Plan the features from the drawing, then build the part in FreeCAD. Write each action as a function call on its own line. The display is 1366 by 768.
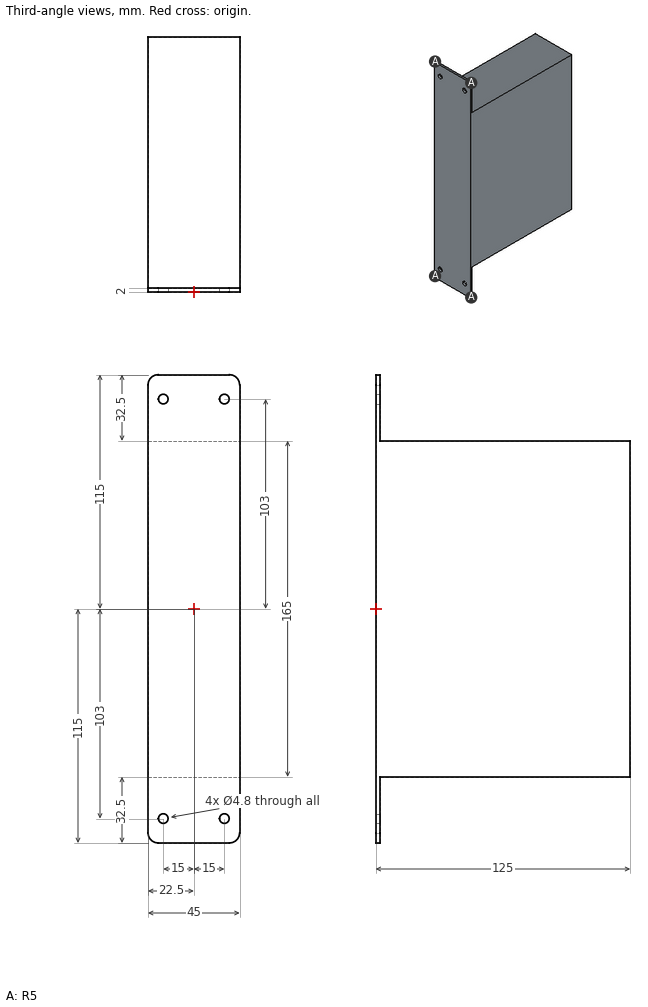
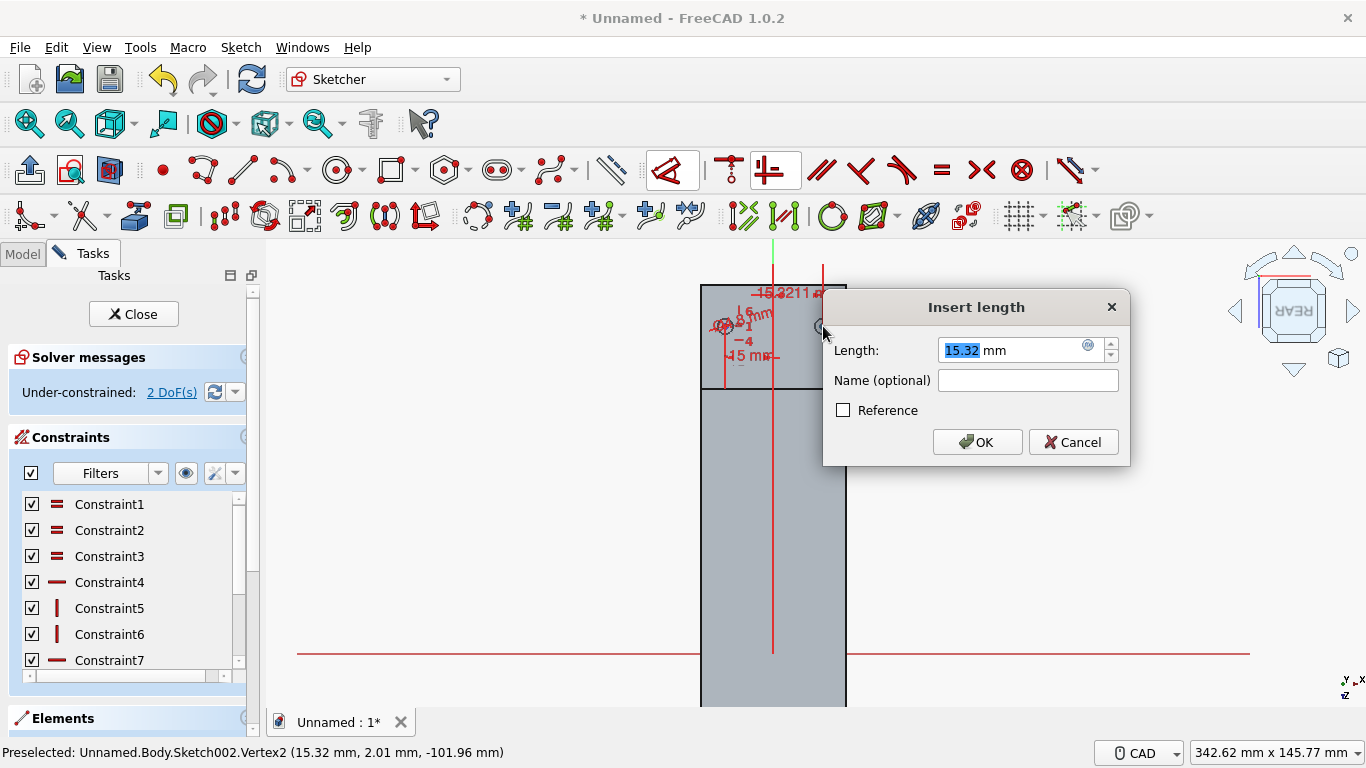
text(15)
key(Return)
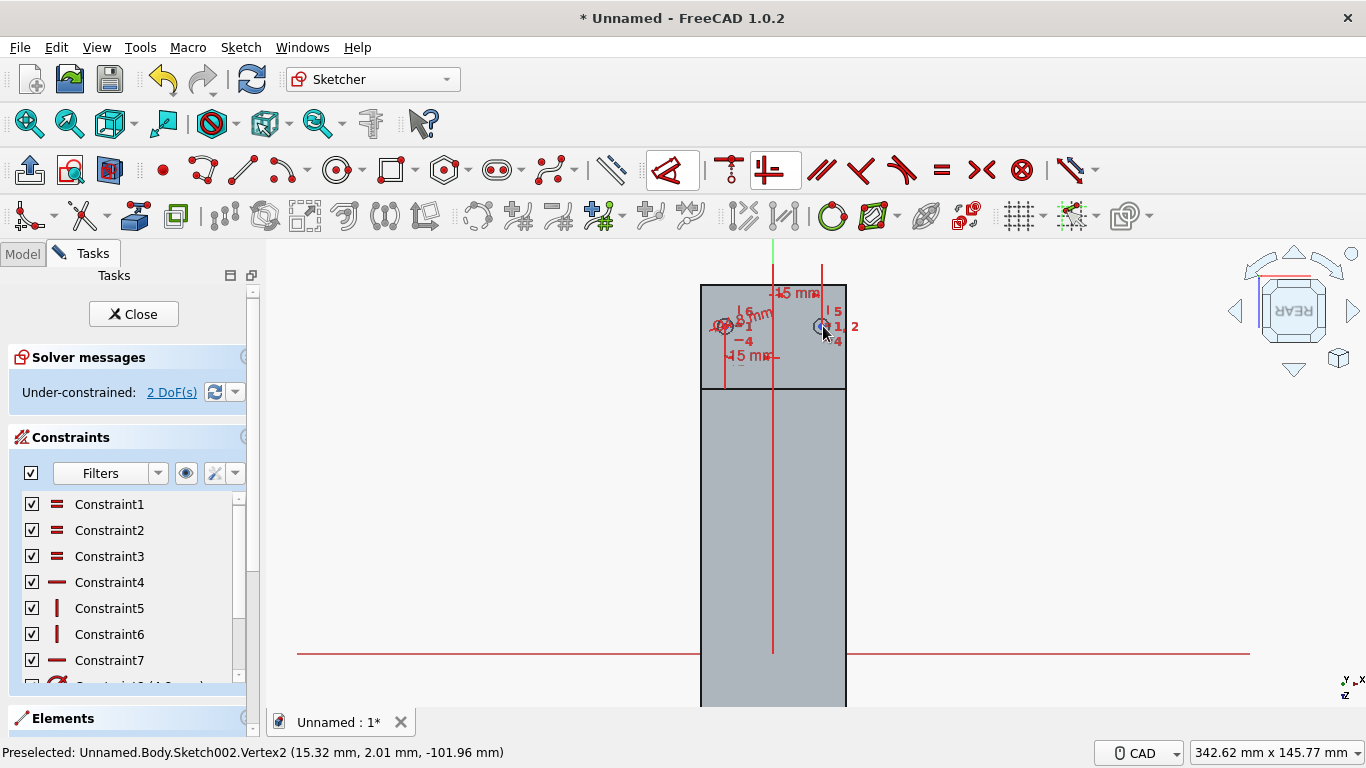
click(725, 326)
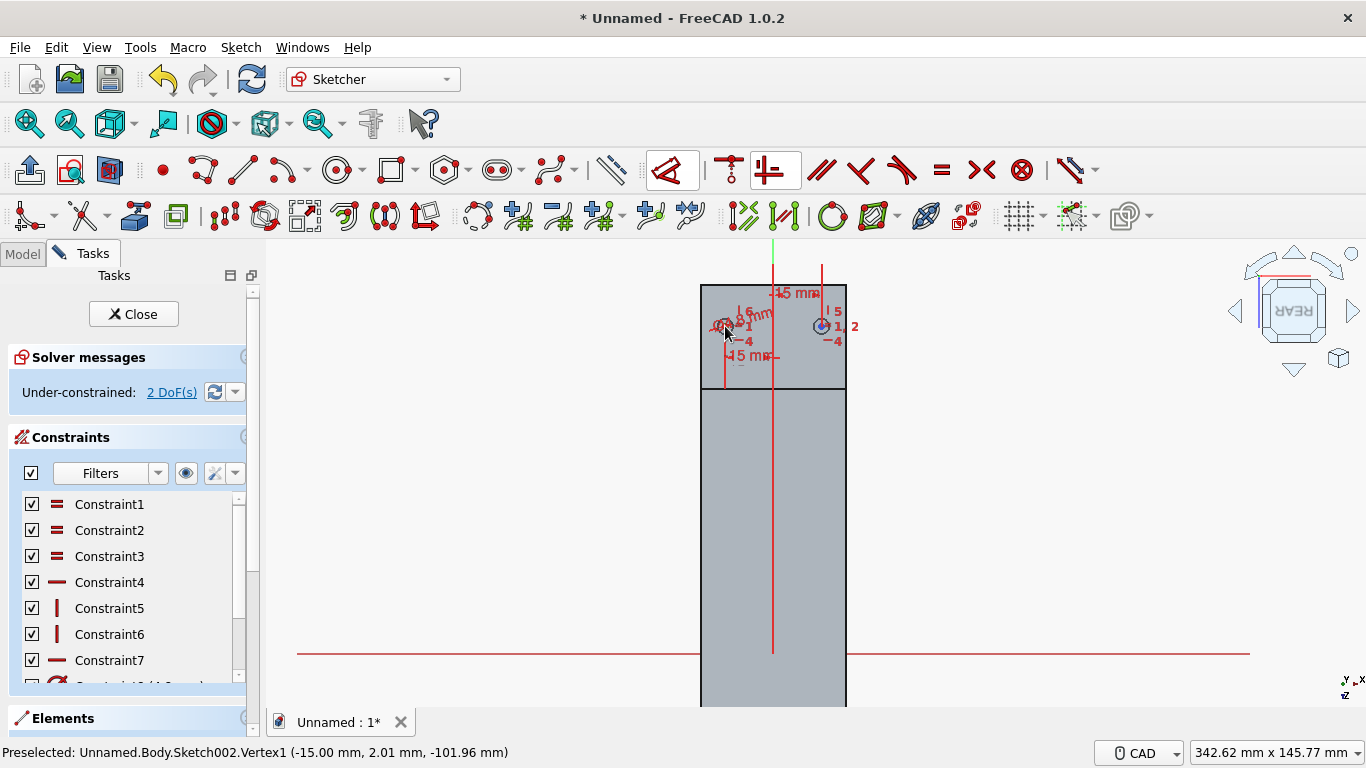
click(694, 170)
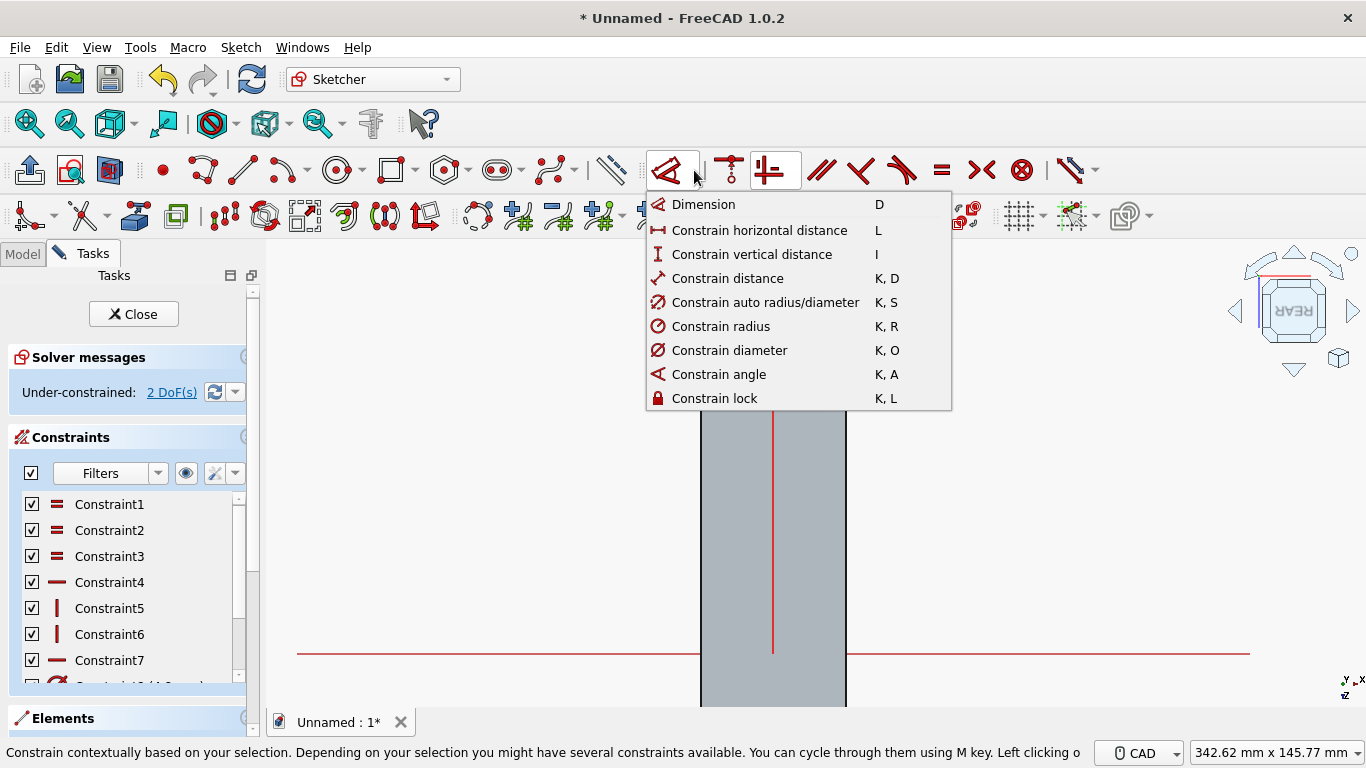
click(799, 254)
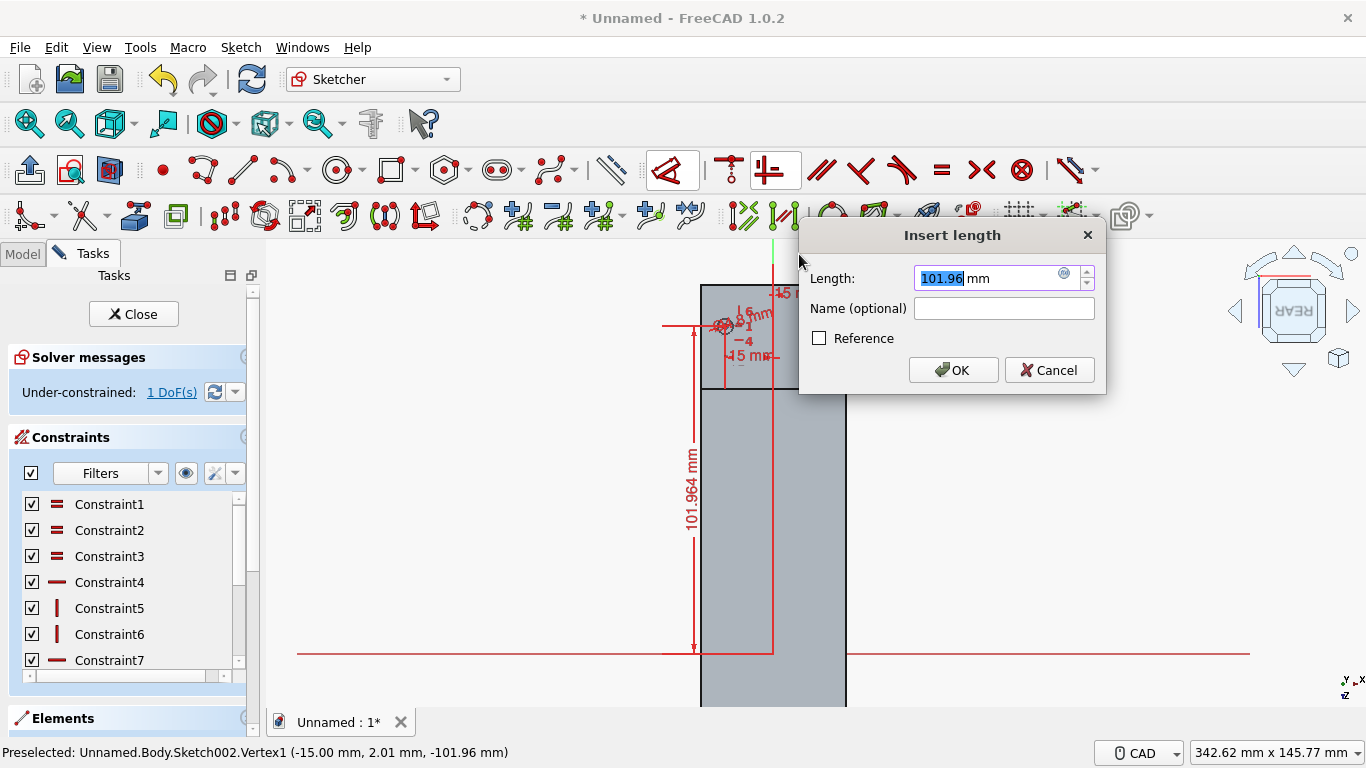
text(103)
key(Return)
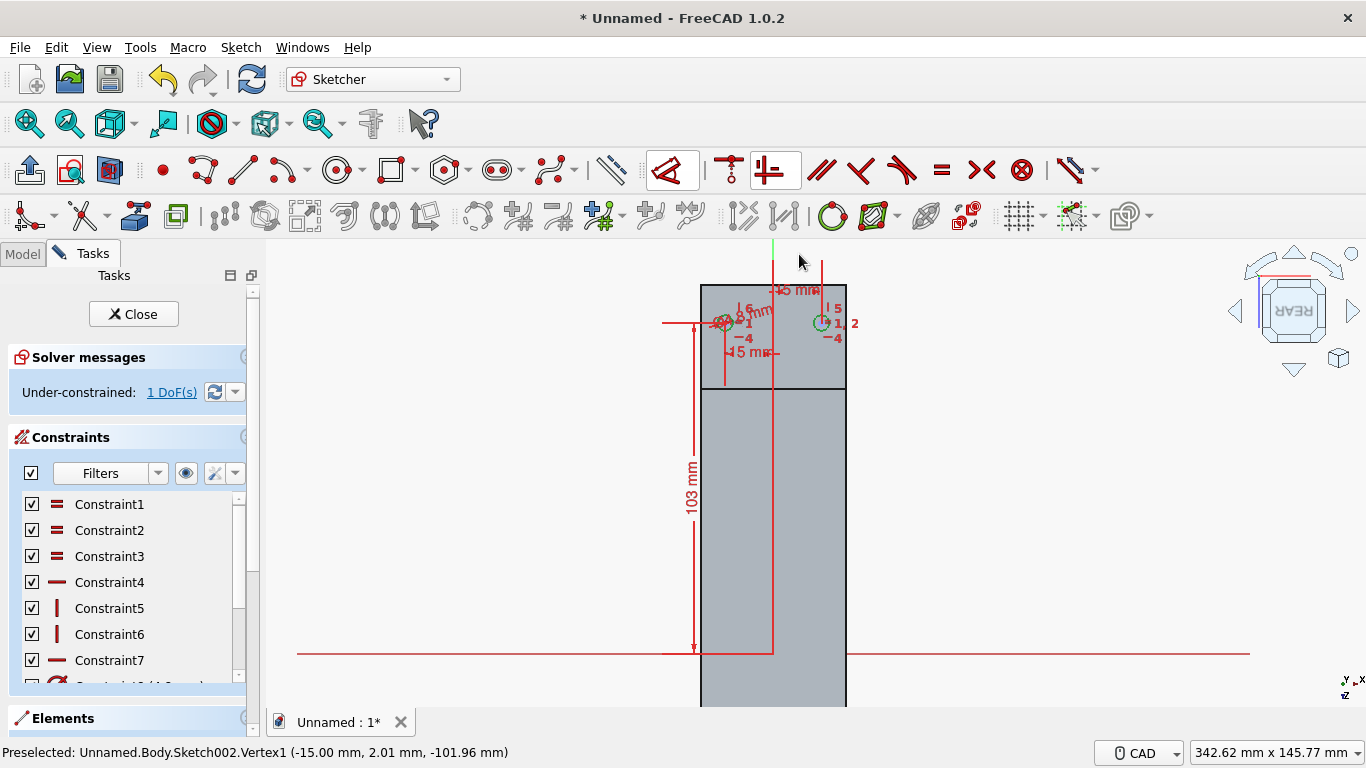
scroll(726, 326, down, 4)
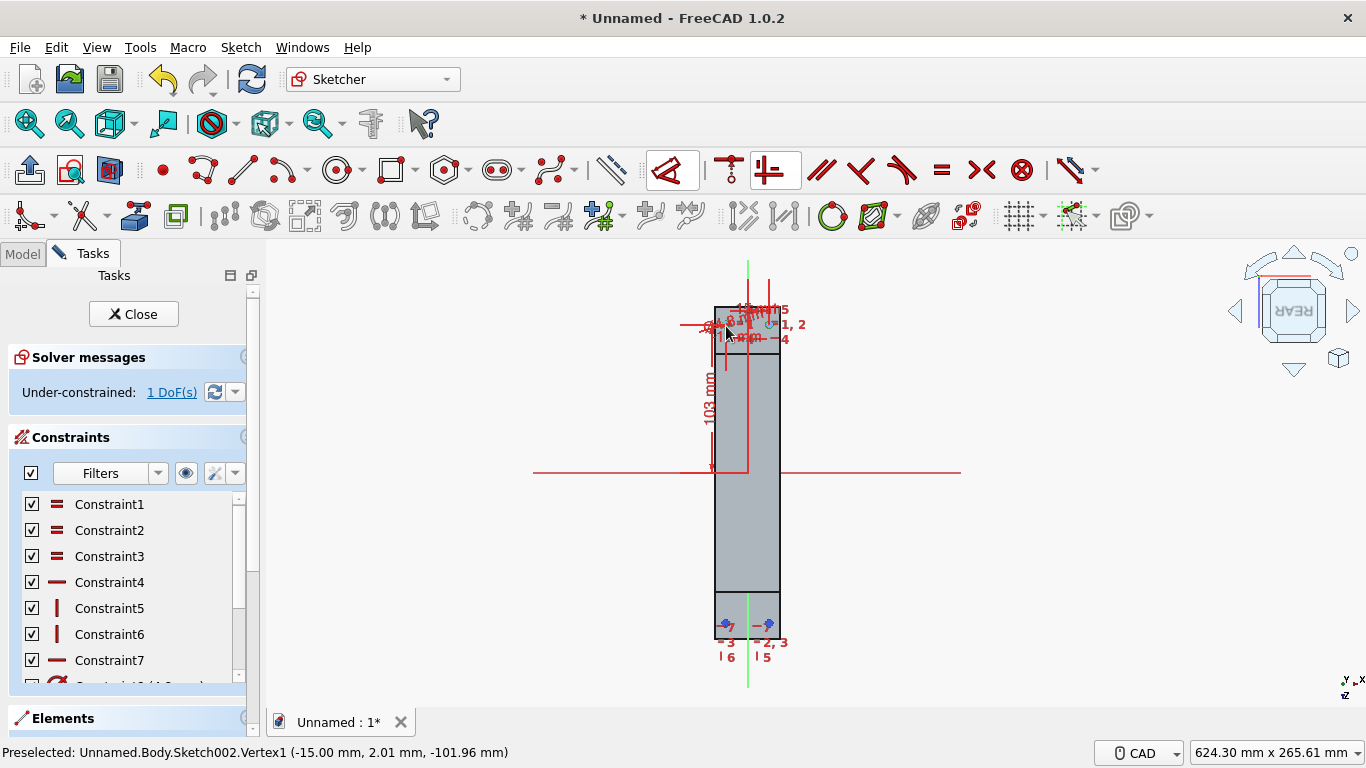
click(769, 623)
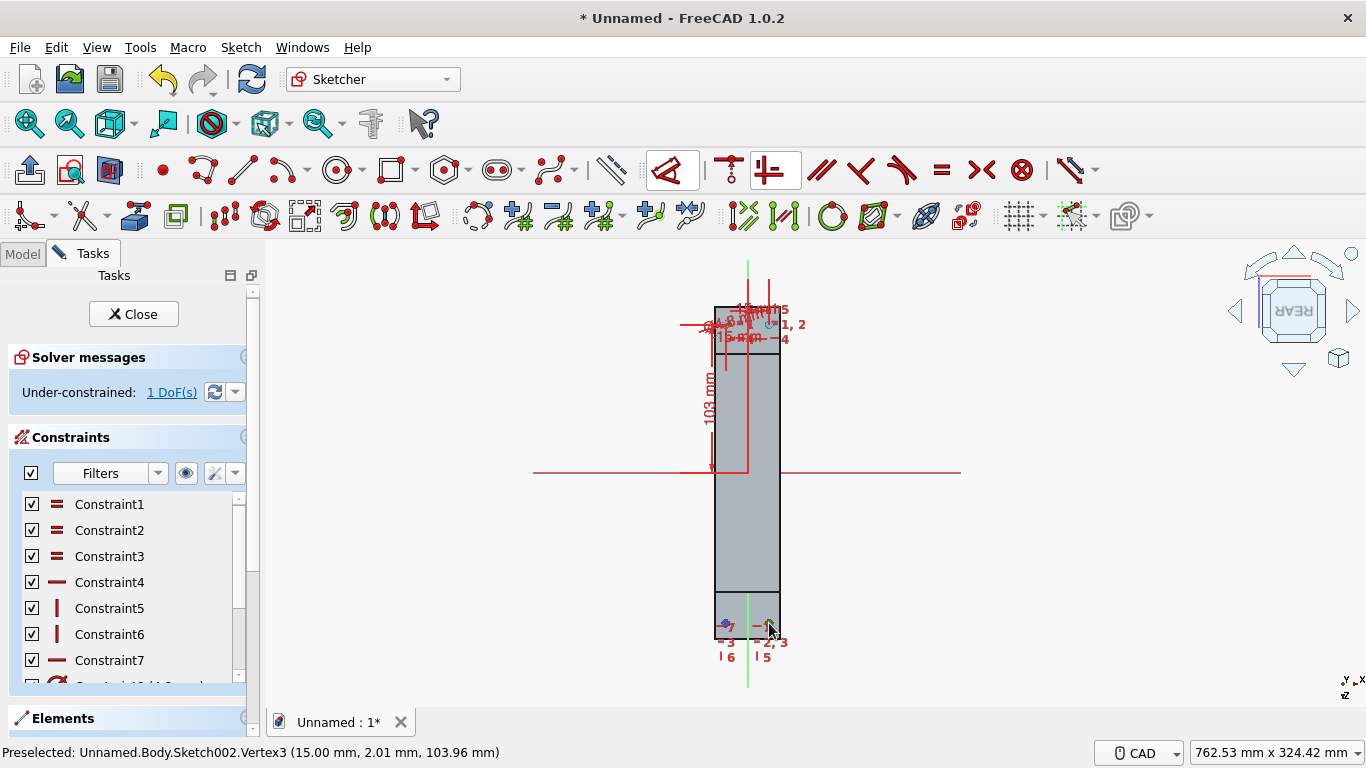
key(i)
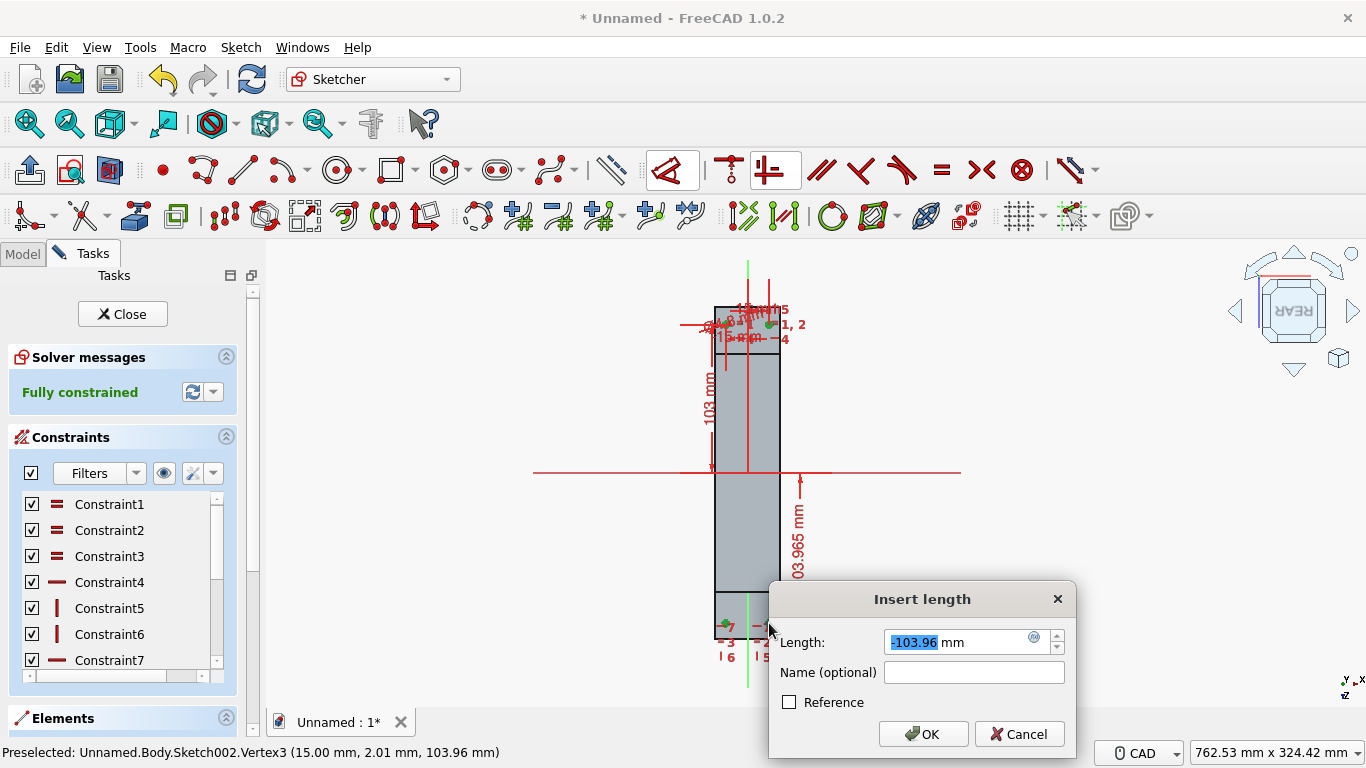
text(-103)
key(Return)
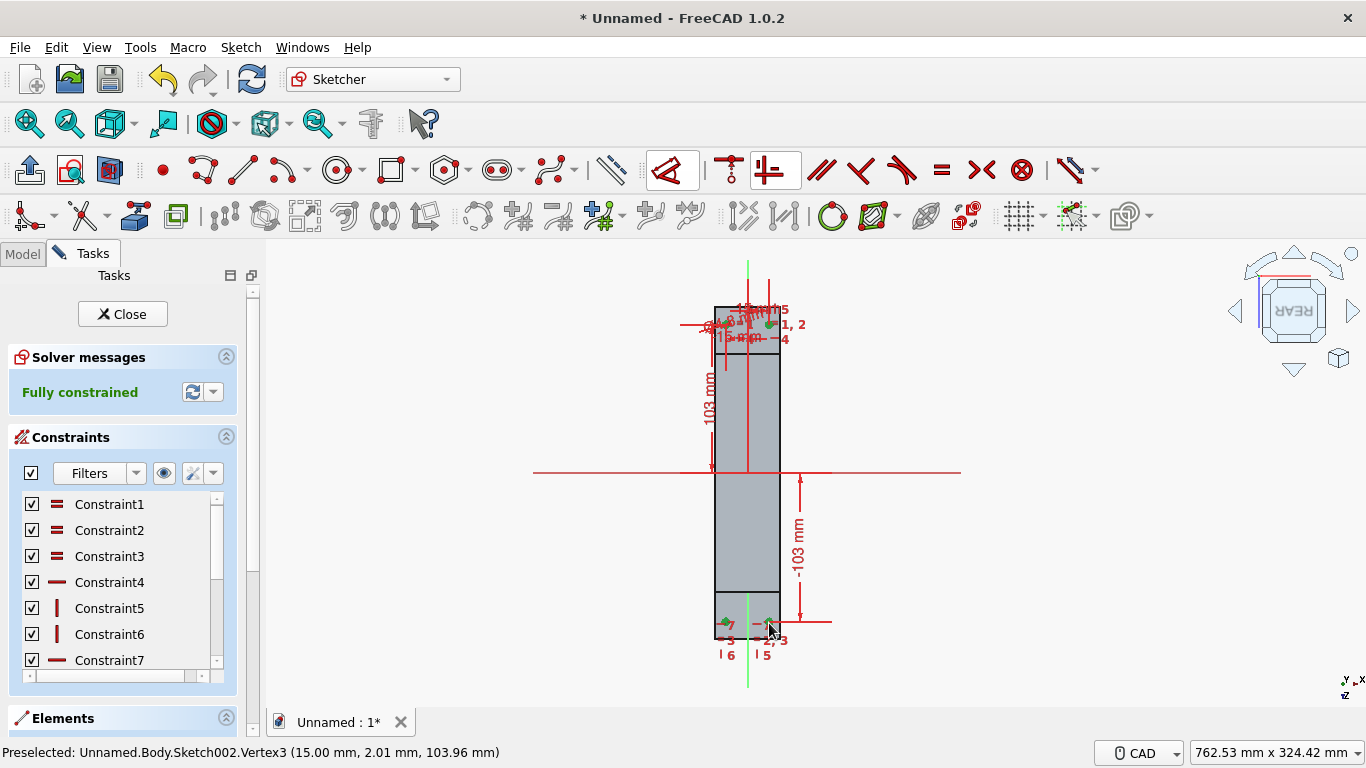
click(123, 314)